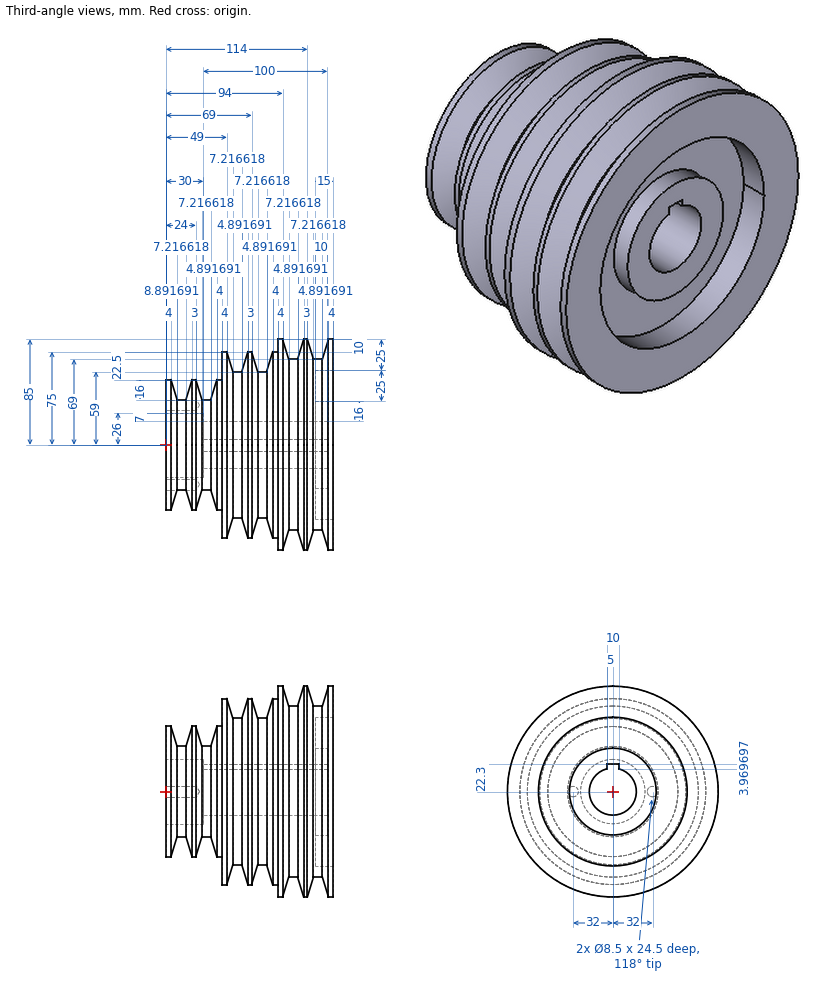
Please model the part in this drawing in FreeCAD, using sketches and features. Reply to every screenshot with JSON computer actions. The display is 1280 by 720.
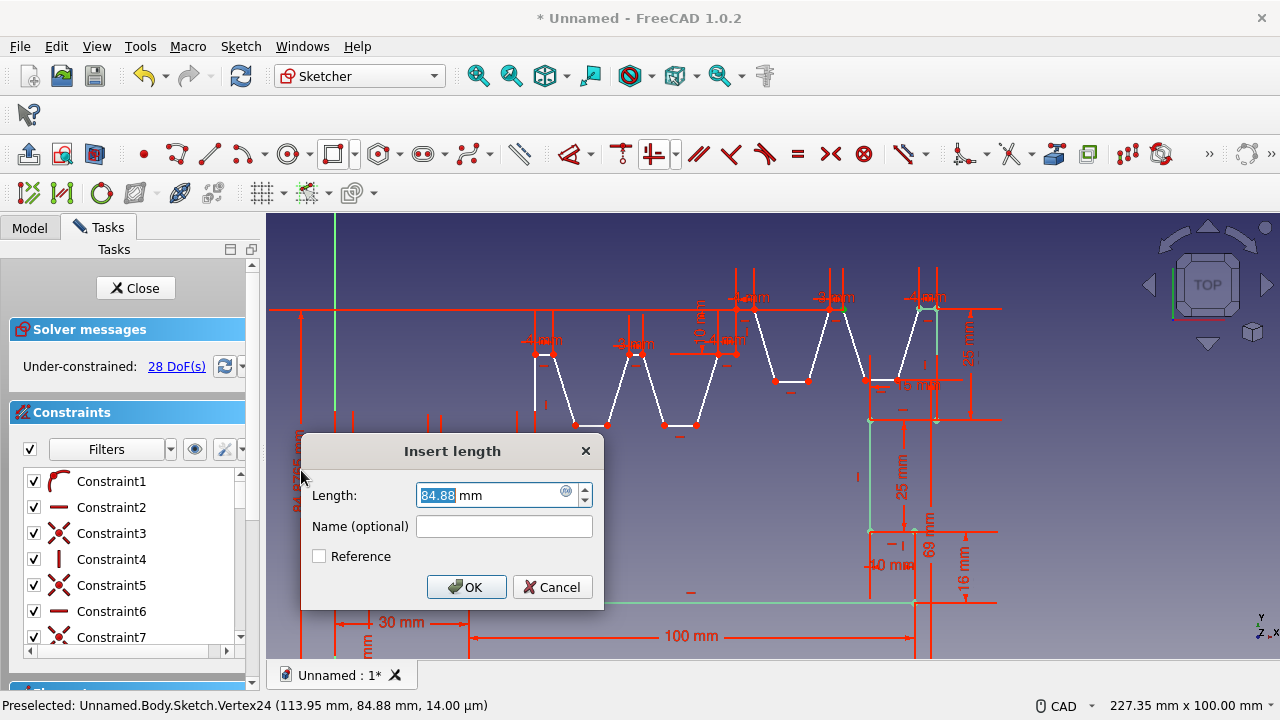
{"action": "type", "text": "85"}
{"action": "key", "text": "Return"}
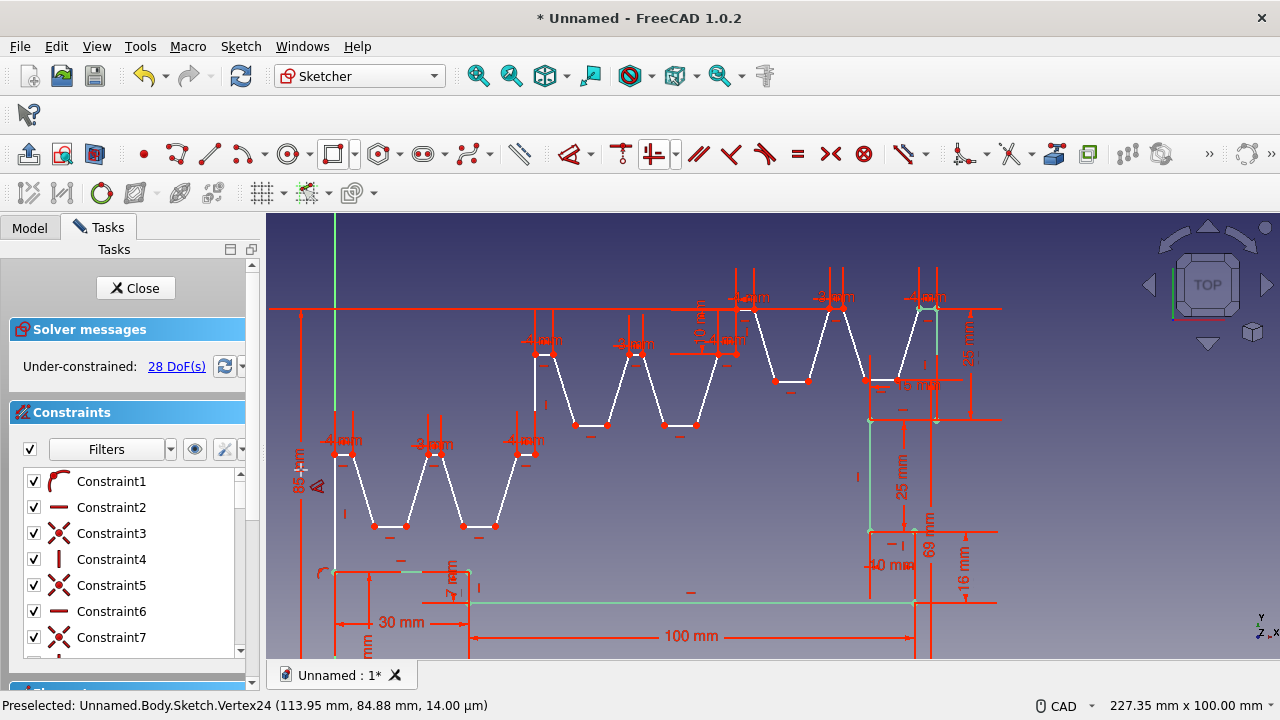
{"action": "left_click", "coordinate": [808, 382]}
{"action": "left_click", "coordinate": [301, 506]}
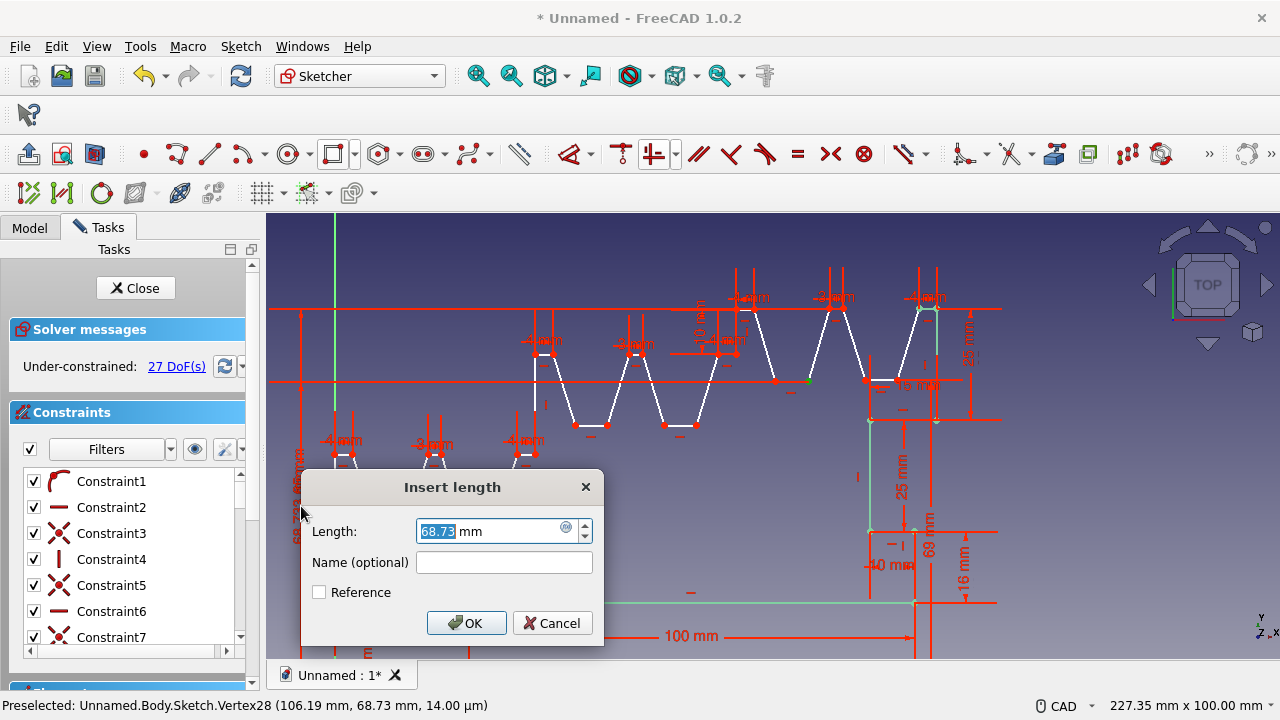
{"action": "type", "text": "69"}
{"action": "key", "text": "Return"}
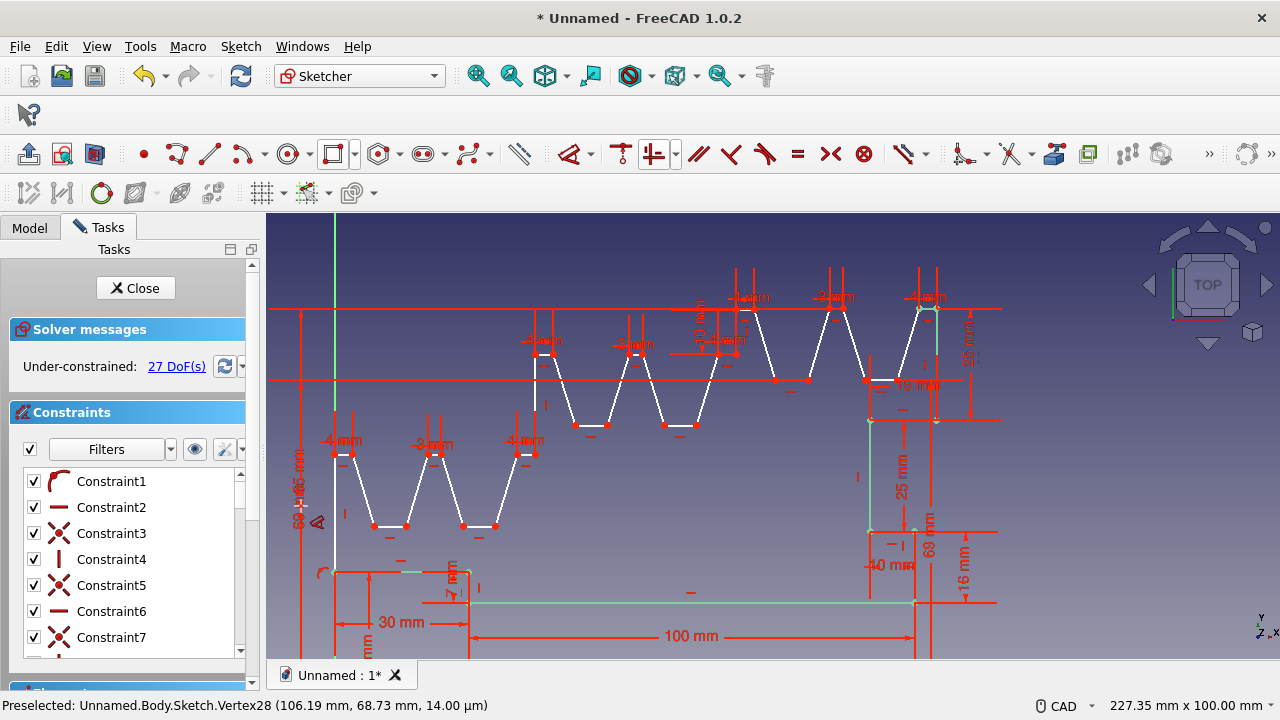
{"action": "left_click", "coordinate": [754, 310]}
{"action": "left_click", "coordinate": [544, 276]}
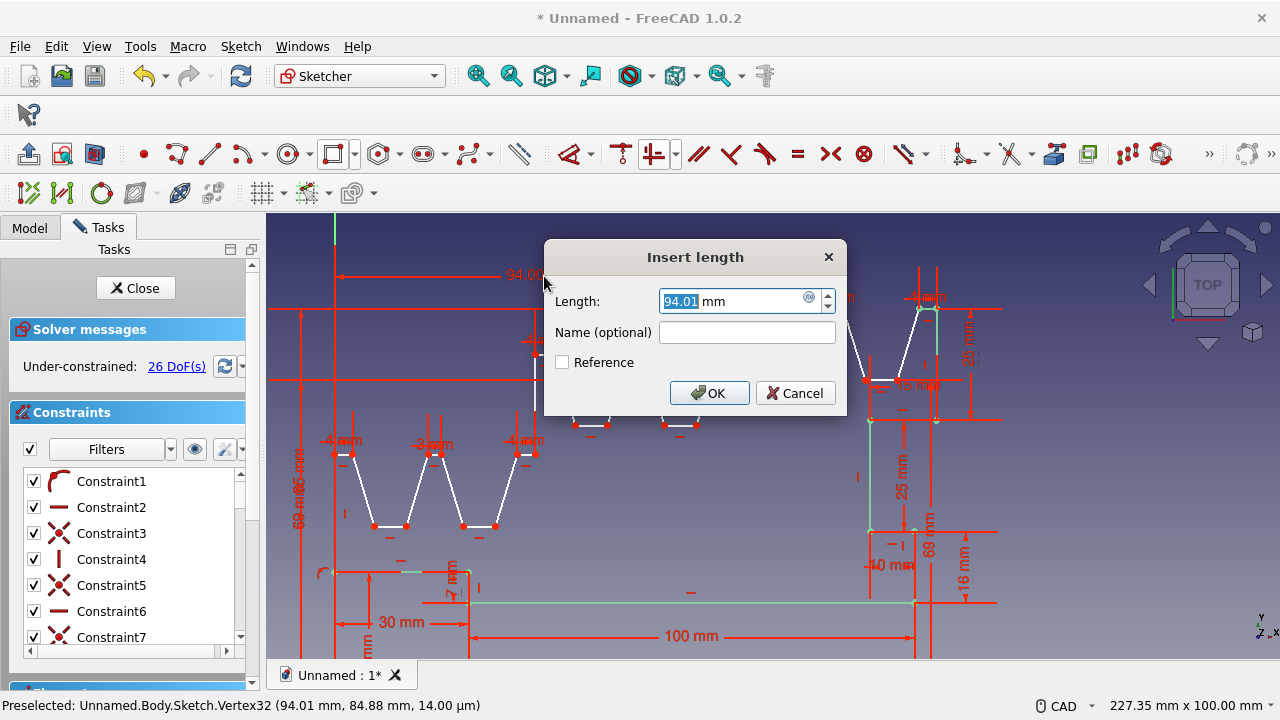
{"action": "type", "text": "94"}
{"action": "key", "text": "Return"}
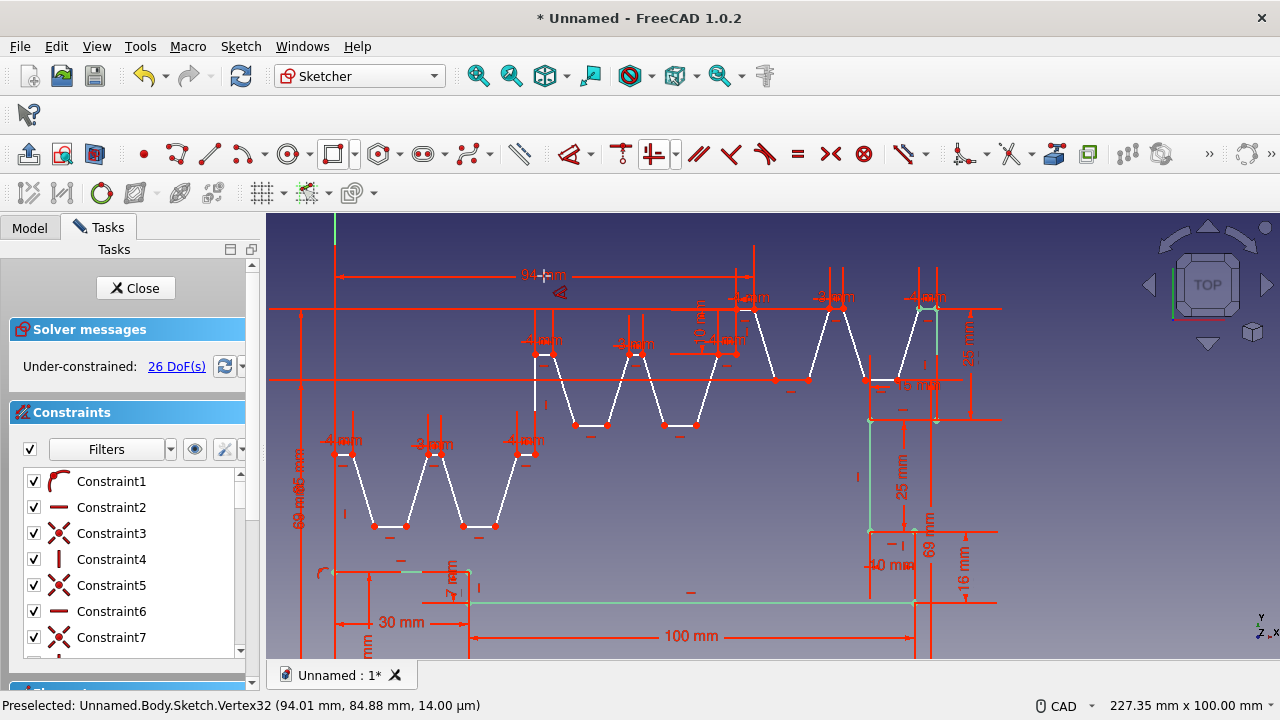
{"action": "left_click", "coordinate": [754, 310]}
{"action": "left_click", "coordinate": [301, 396]}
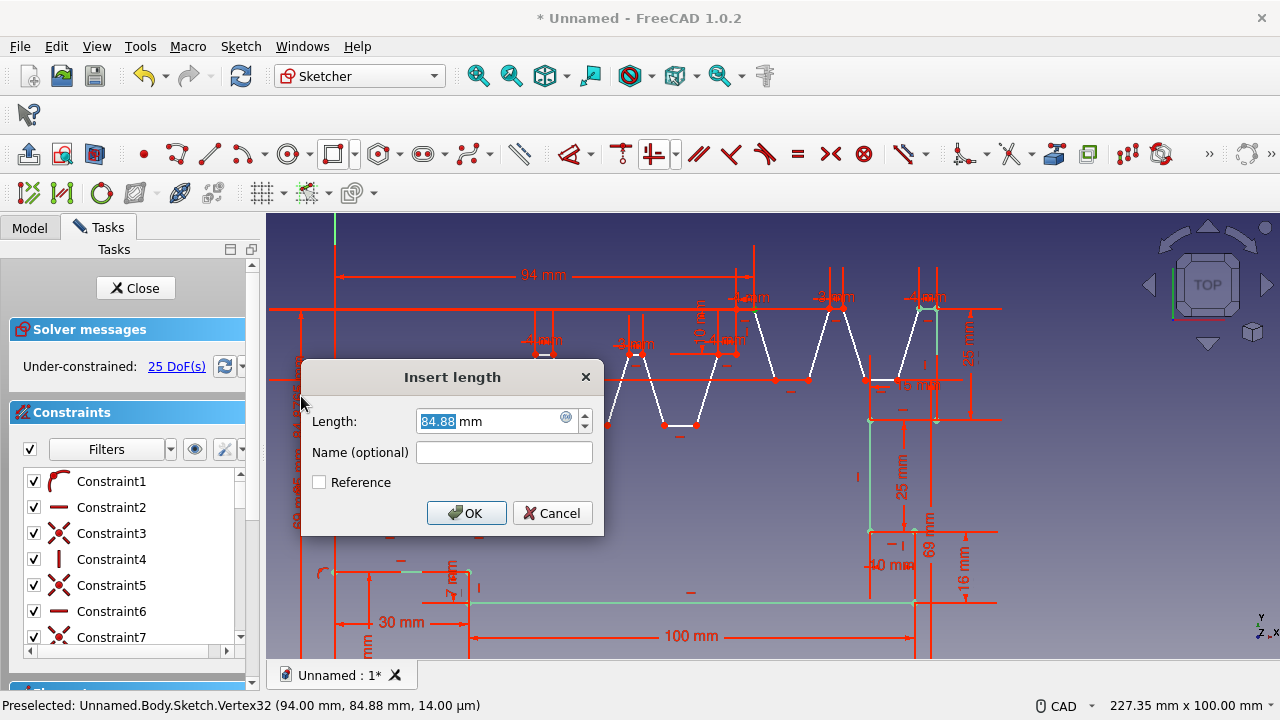
{"action": "type", "text": "85"}
{"action": "key", "text": "Return"}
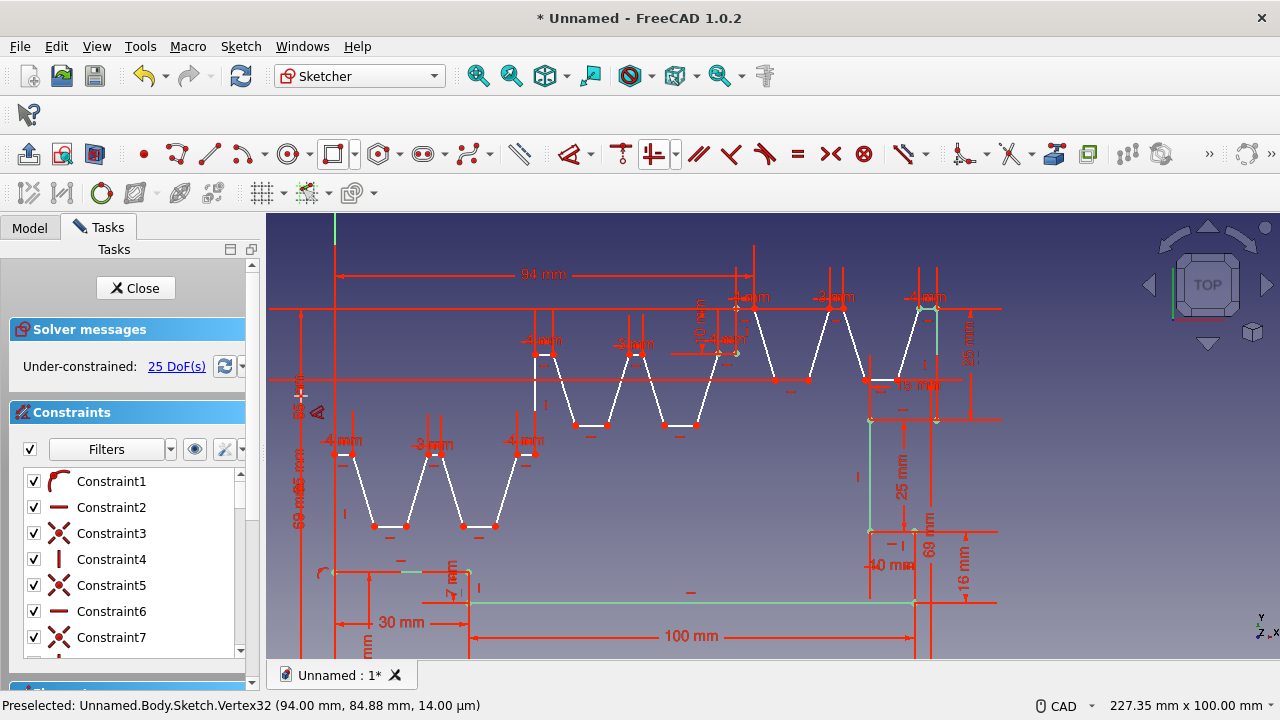
{"action": "left_click", "coordinate": [696, 426]}
{"action": "left_click", "coordinate": [301, 528]}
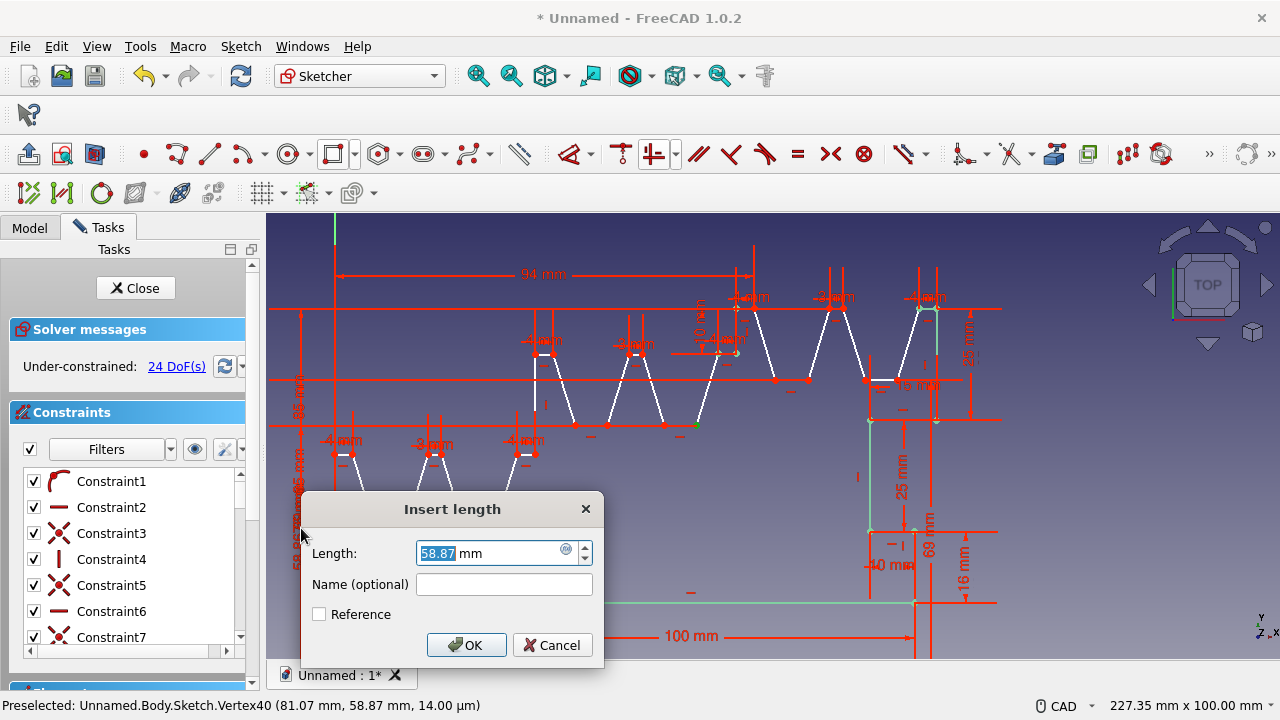
{"action": "type", "text": "59"}
{"action": "key", "text": "Return"}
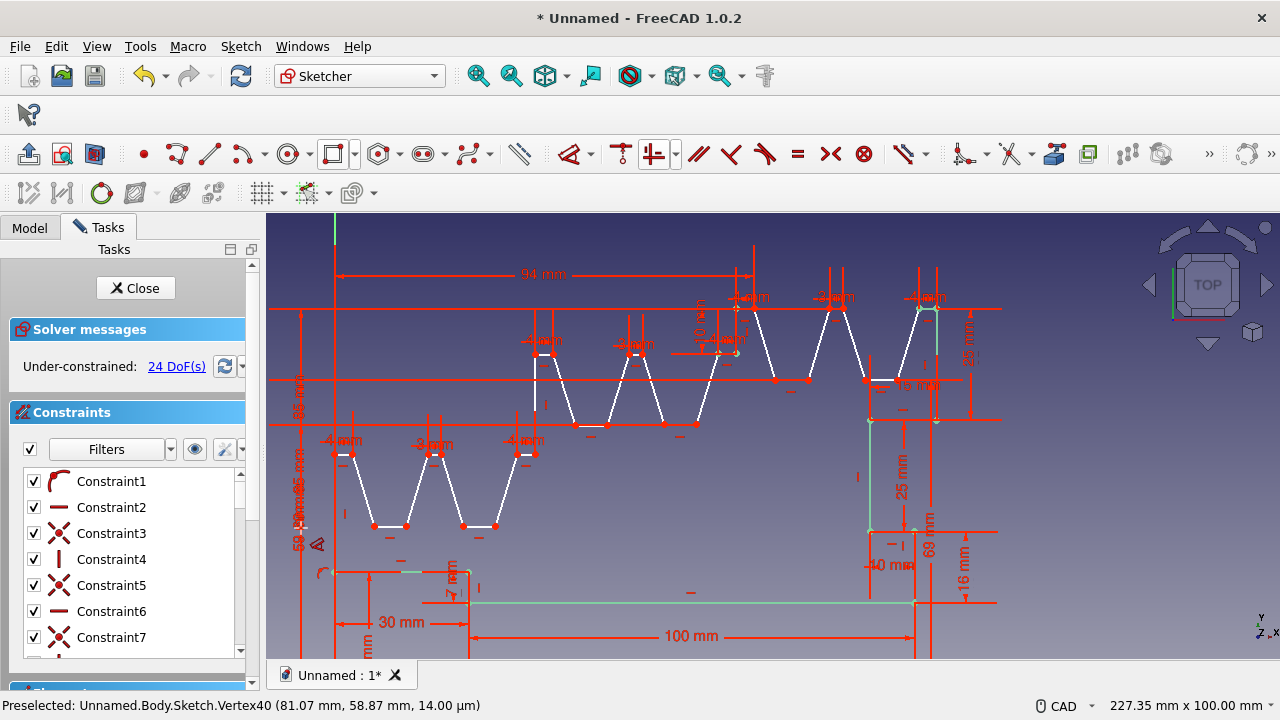
{"action": "left_click", "coordinate": [643, 355]}
{"action": "left_click", "coordinate": [489, 321]}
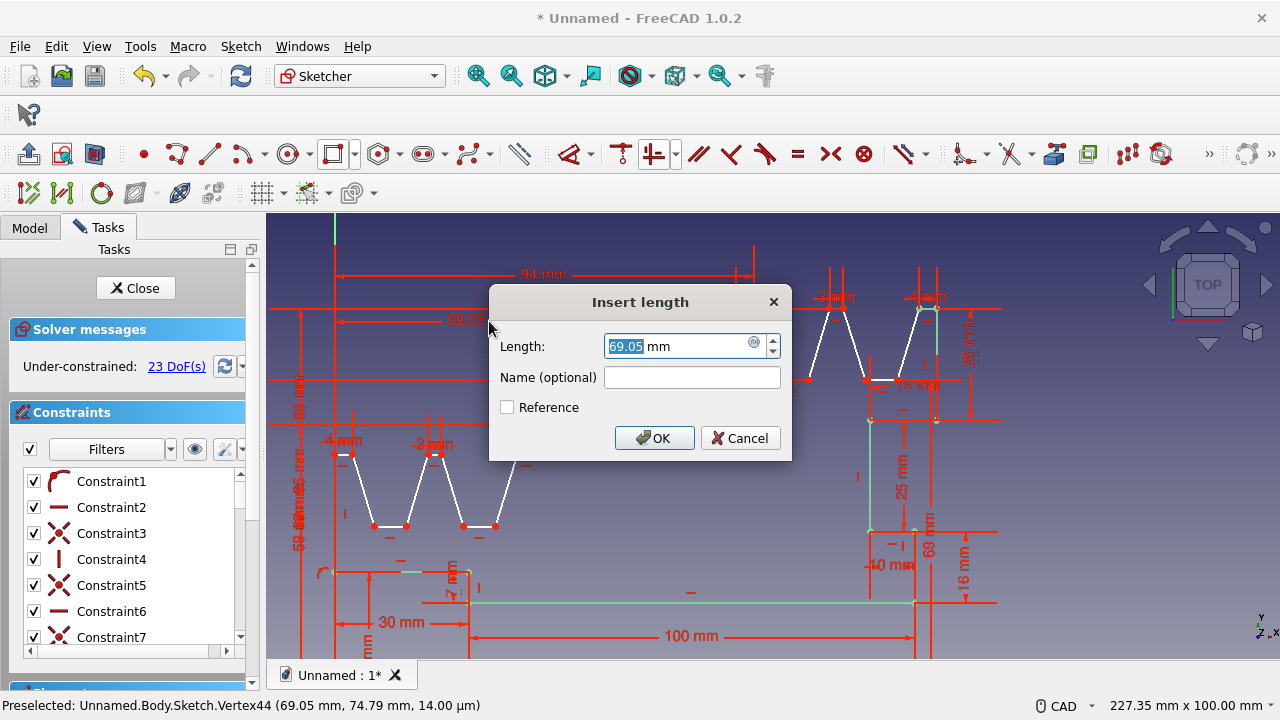
{"action": "type", "text": "69"}
{"action": "key", "text": "Return"}